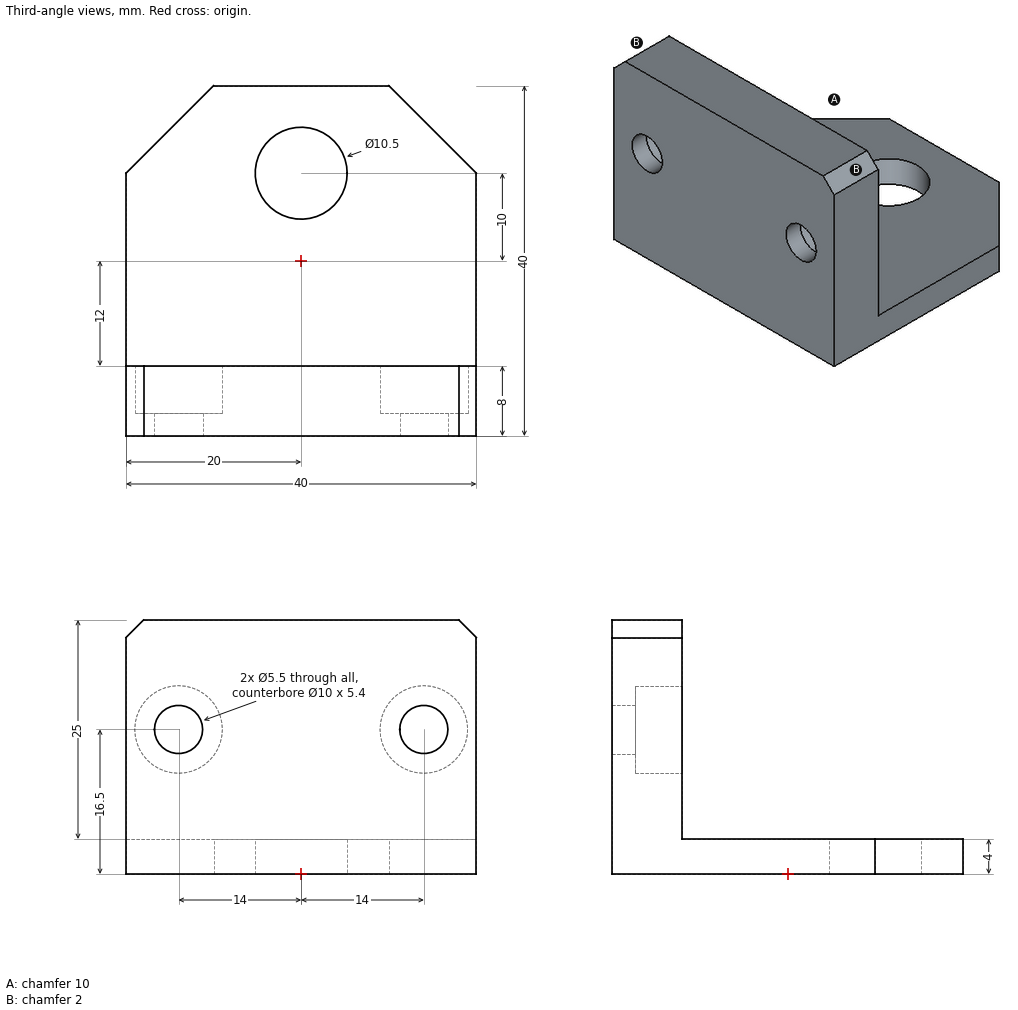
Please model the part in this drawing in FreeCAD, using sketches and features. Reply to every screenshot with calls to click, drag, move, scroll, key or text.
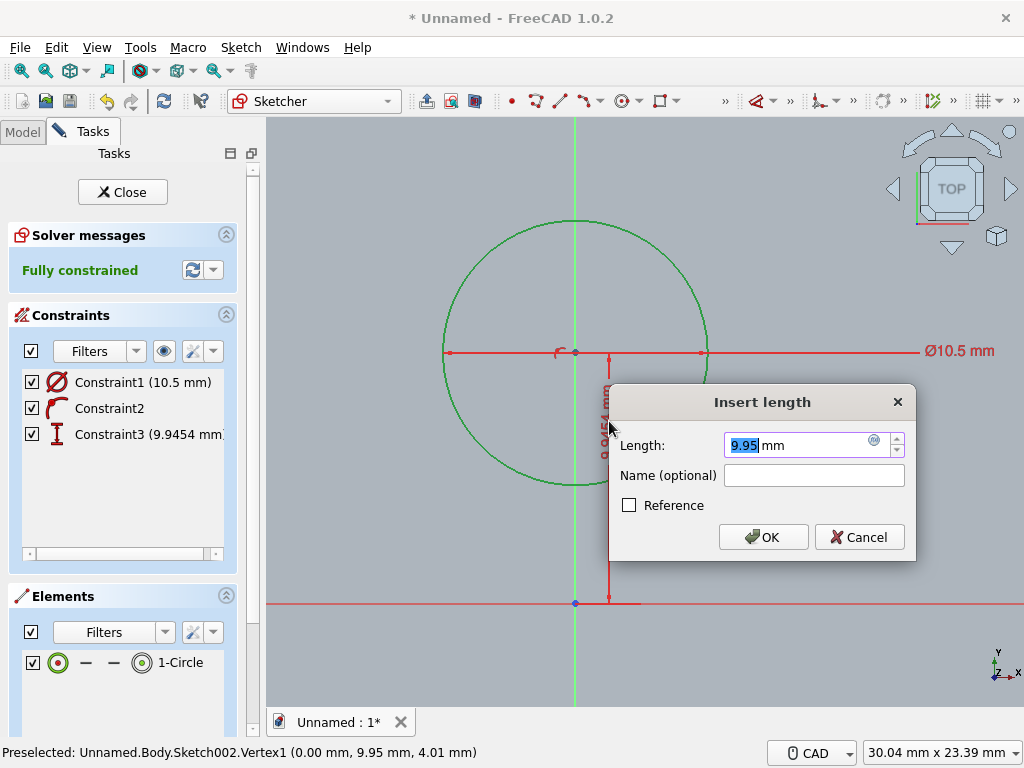
text(10)
key(Return)
key(Escape)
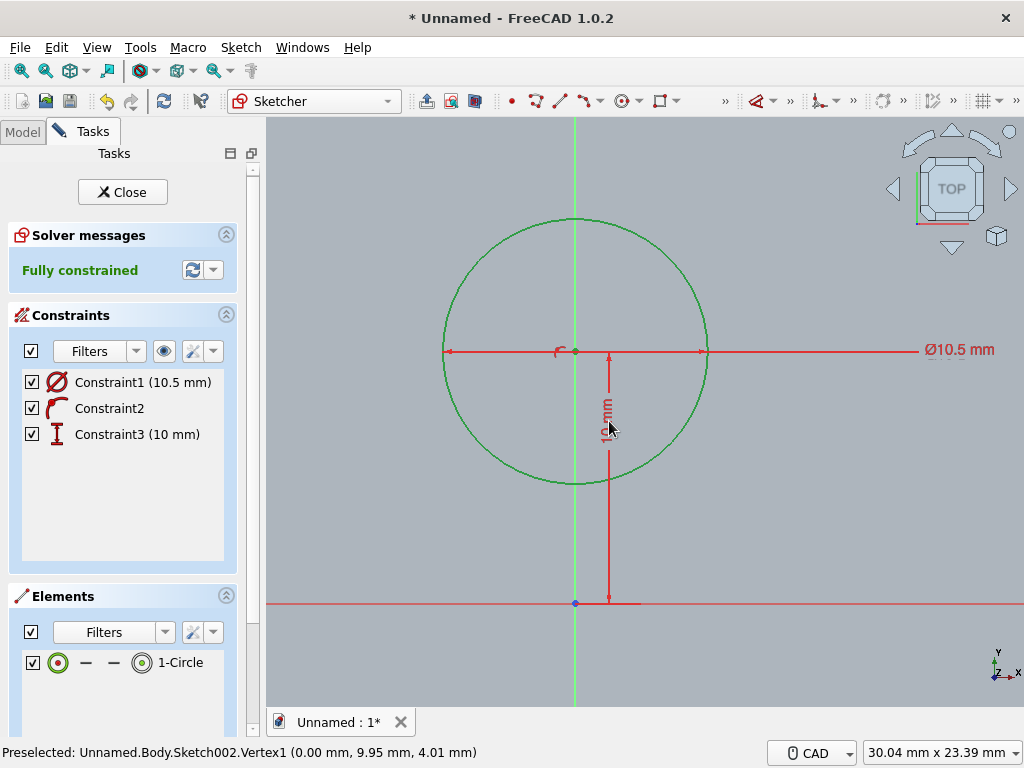
click(123, 192)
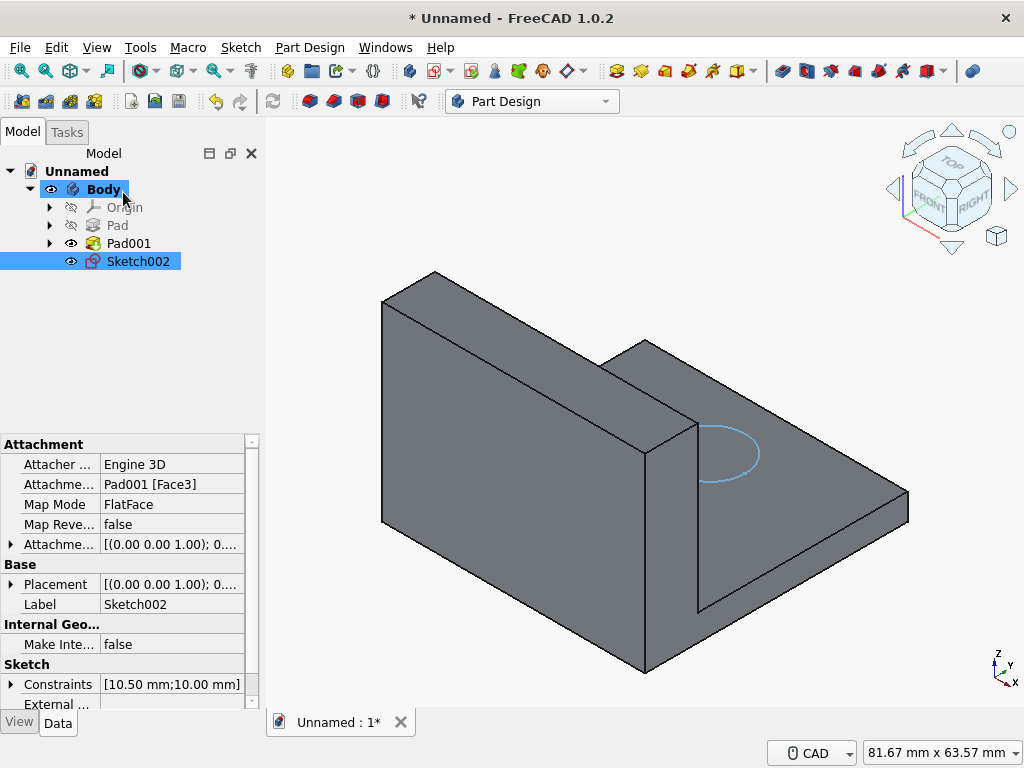
click(784, 72)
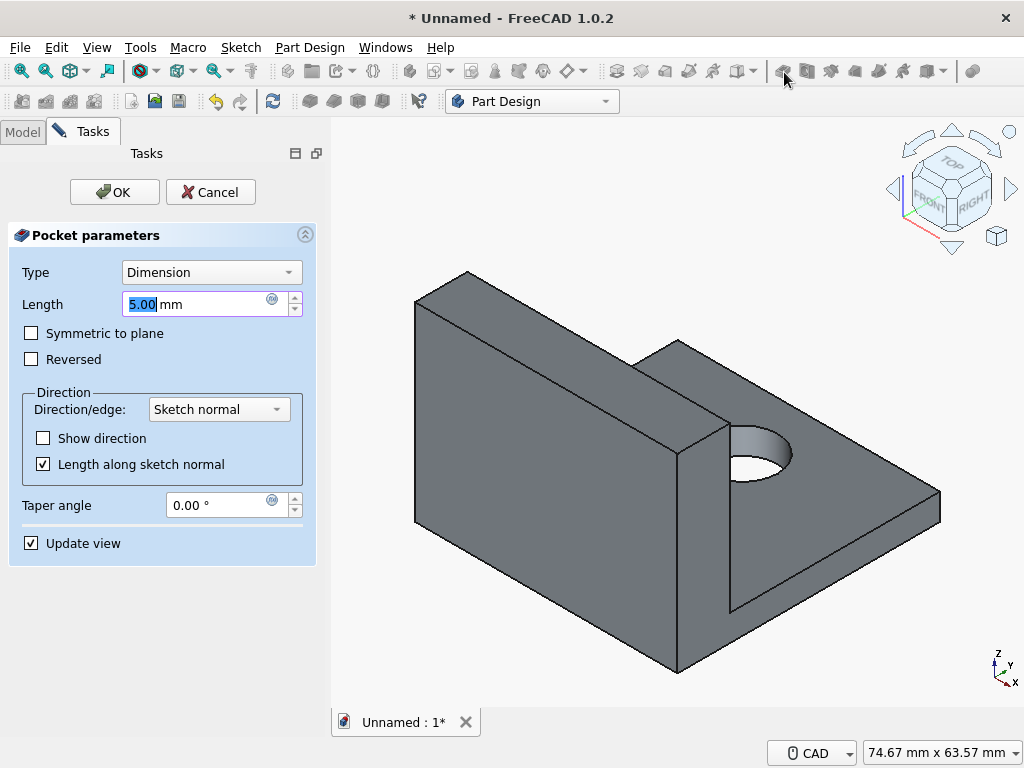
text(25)
key(Tab)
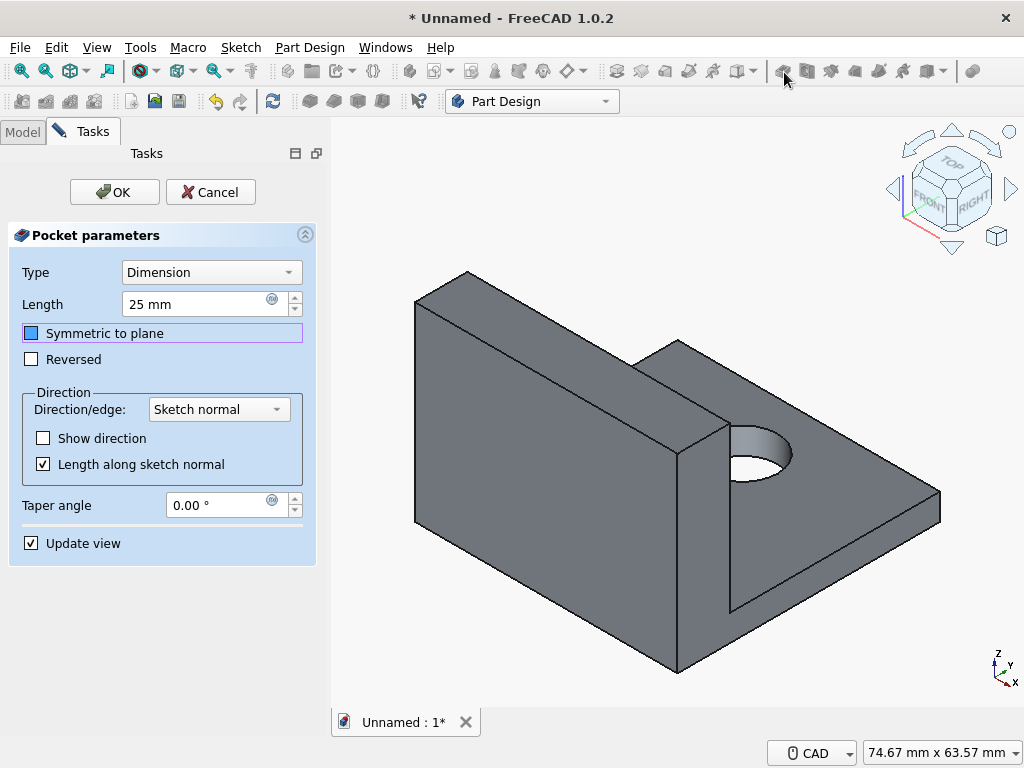
click(115, 192)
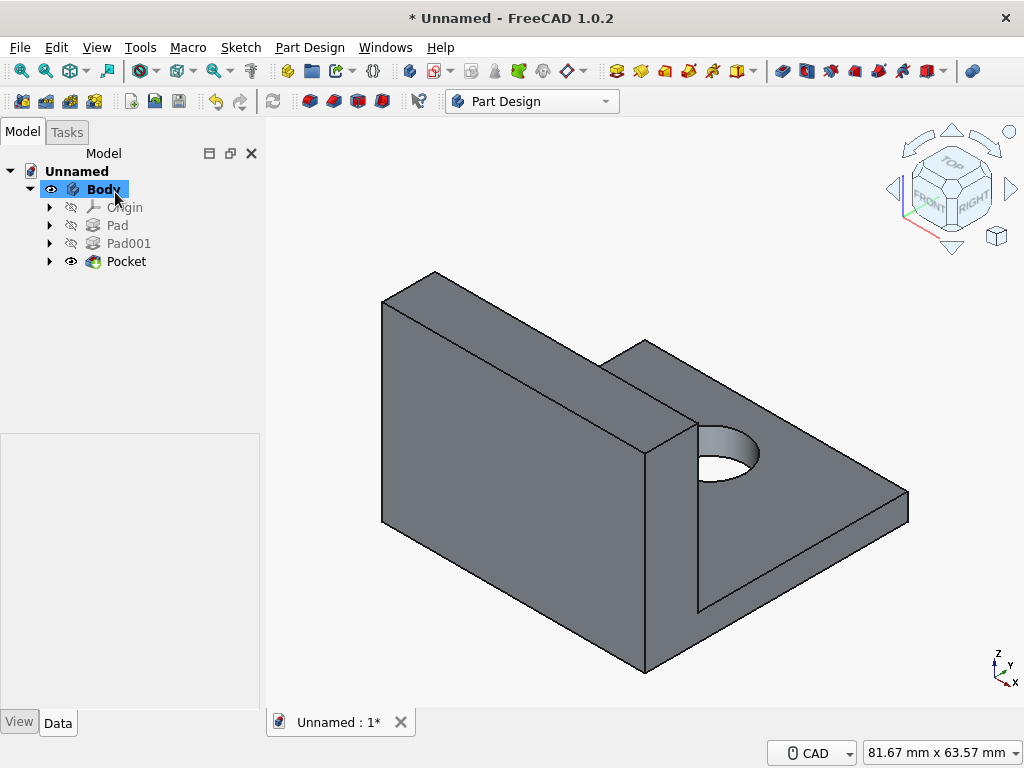
key(2)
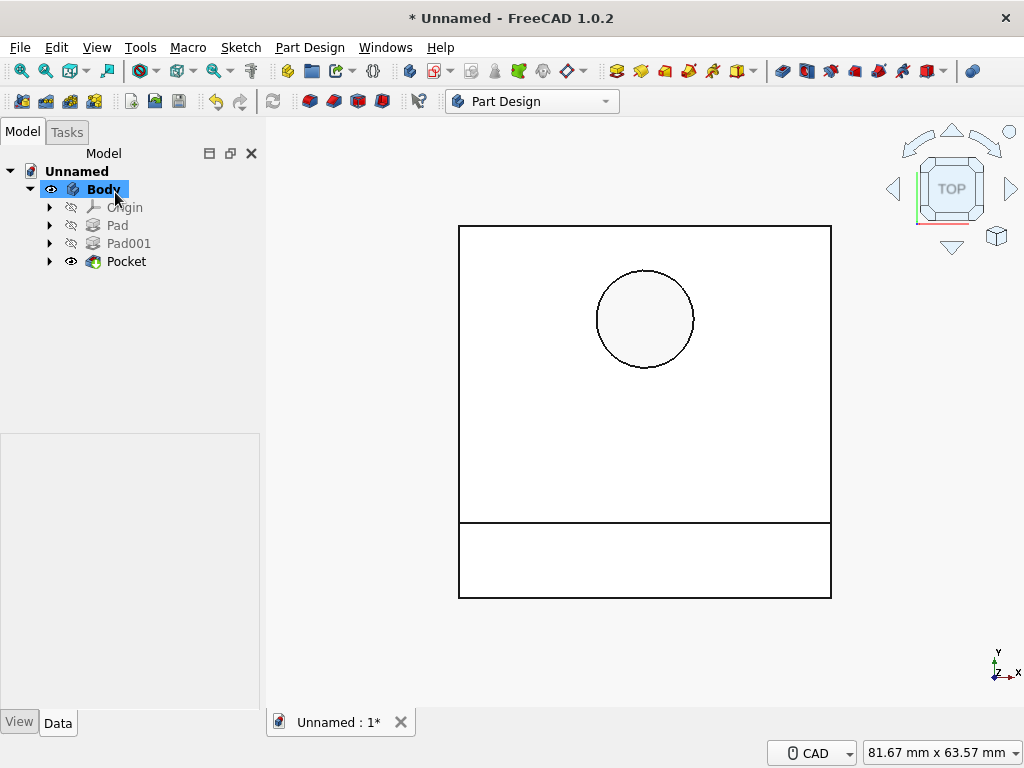
key(0)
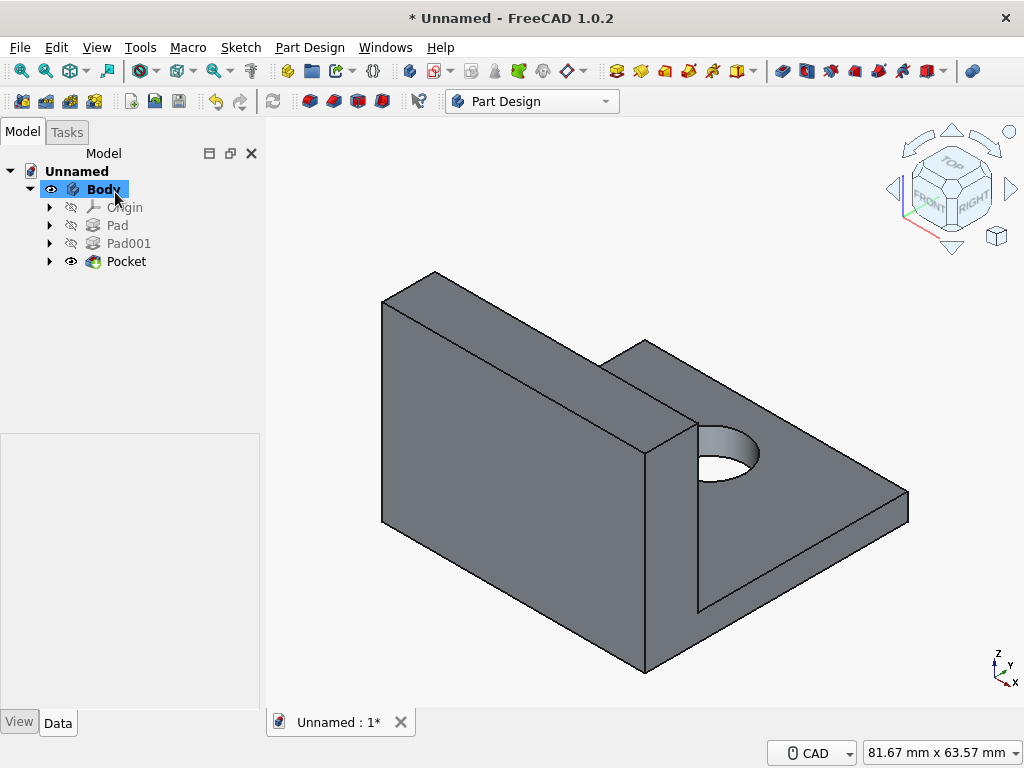
key(1)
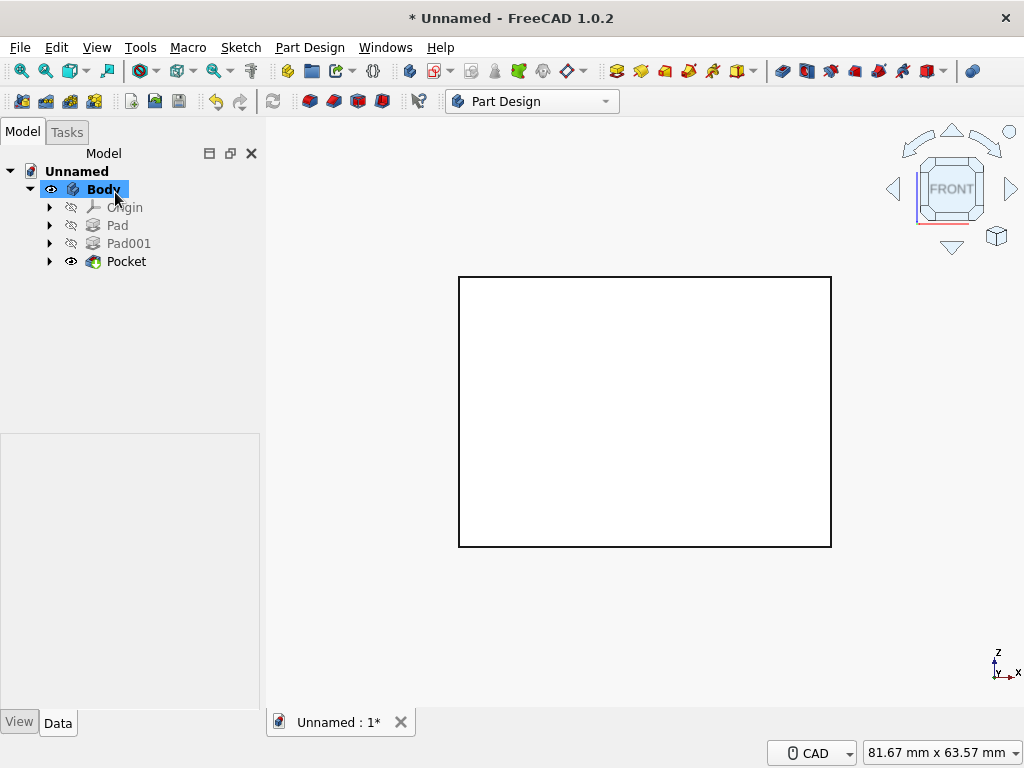
key(3)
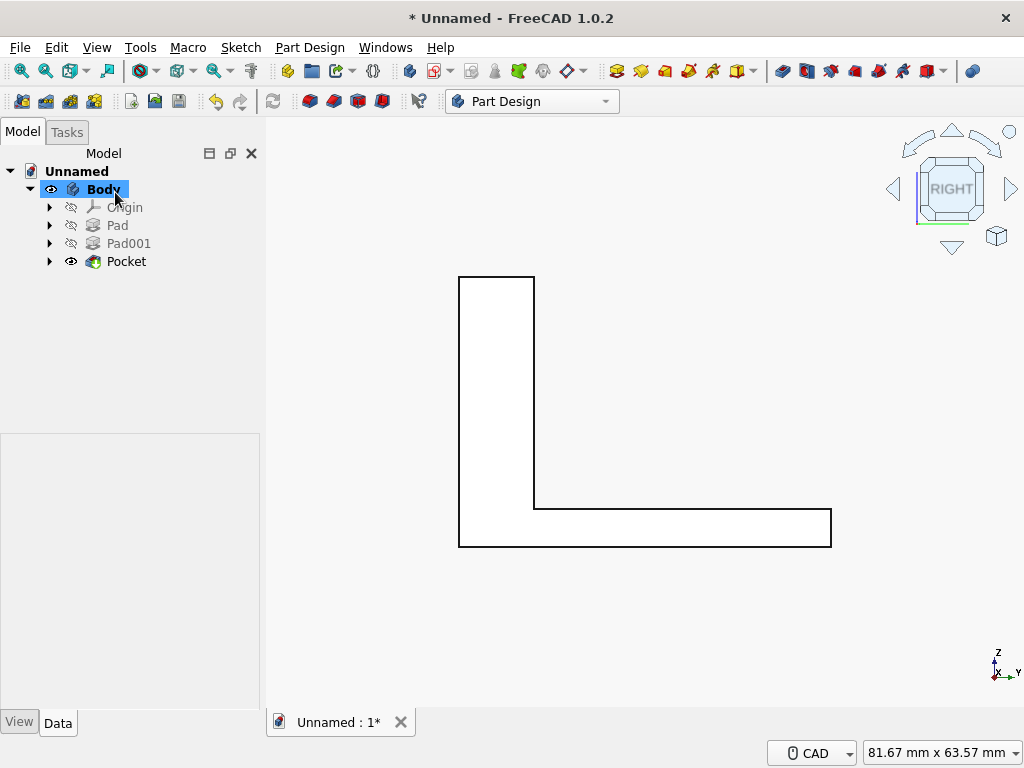
click(831, 527)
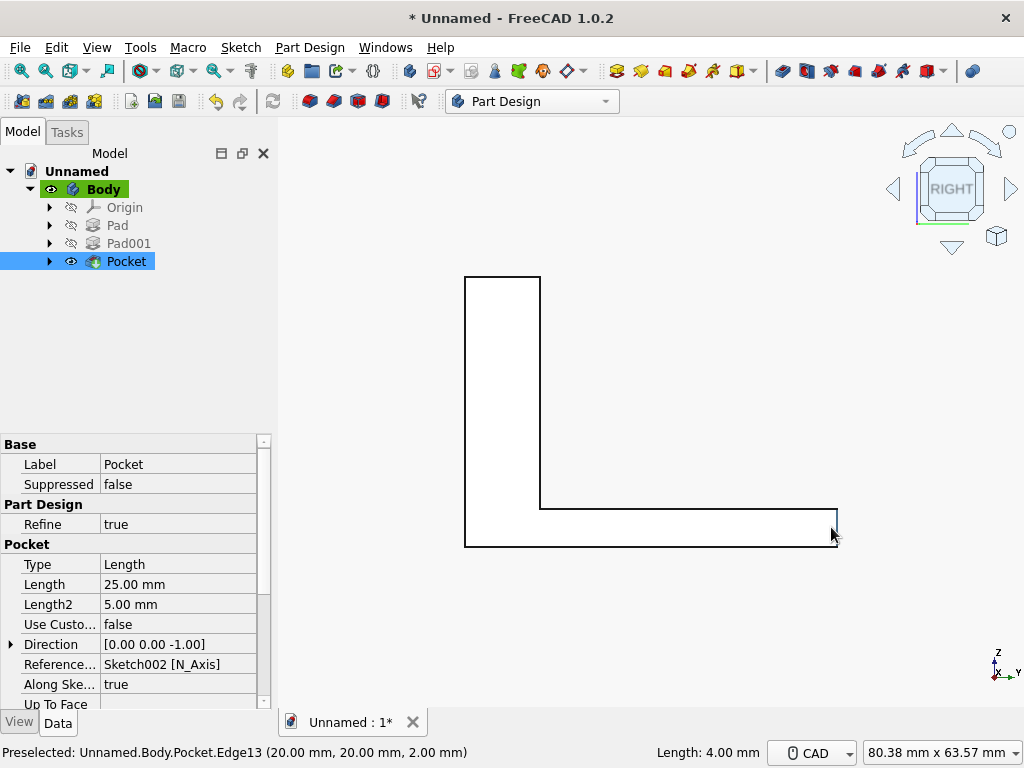
key(5)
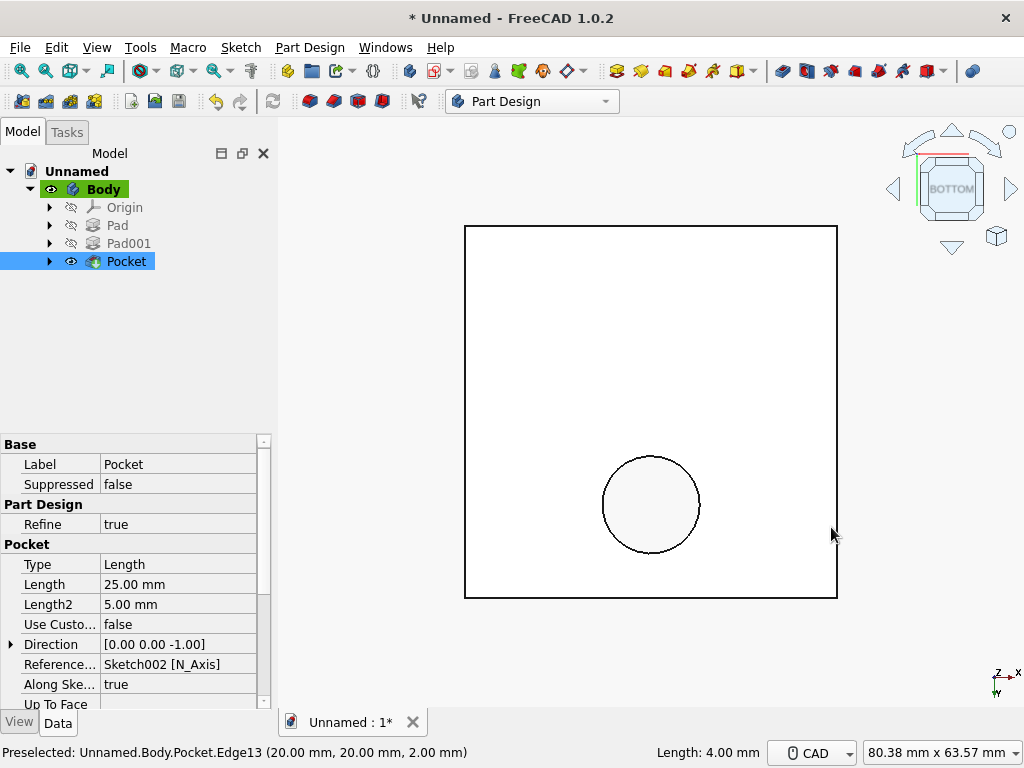
key(4)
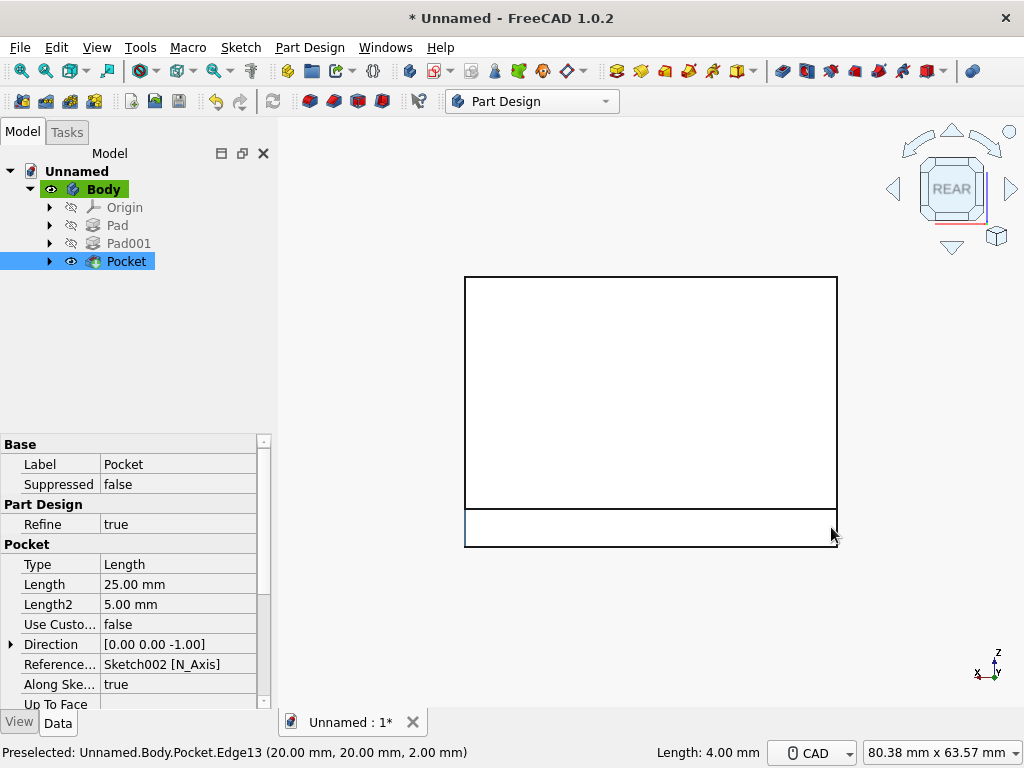
click(837, 527, ctrl)